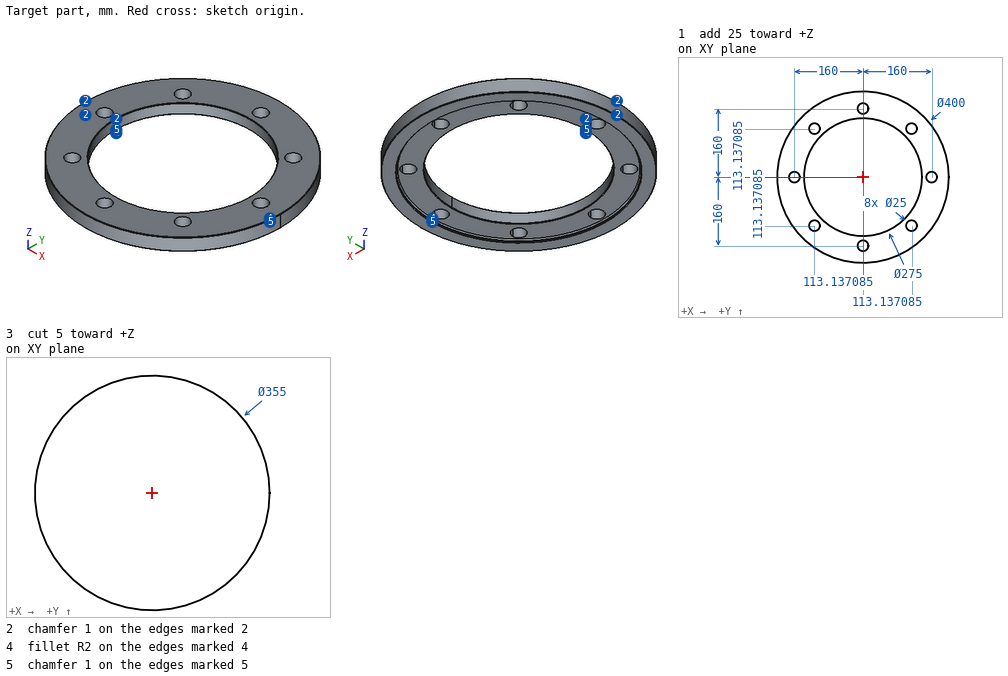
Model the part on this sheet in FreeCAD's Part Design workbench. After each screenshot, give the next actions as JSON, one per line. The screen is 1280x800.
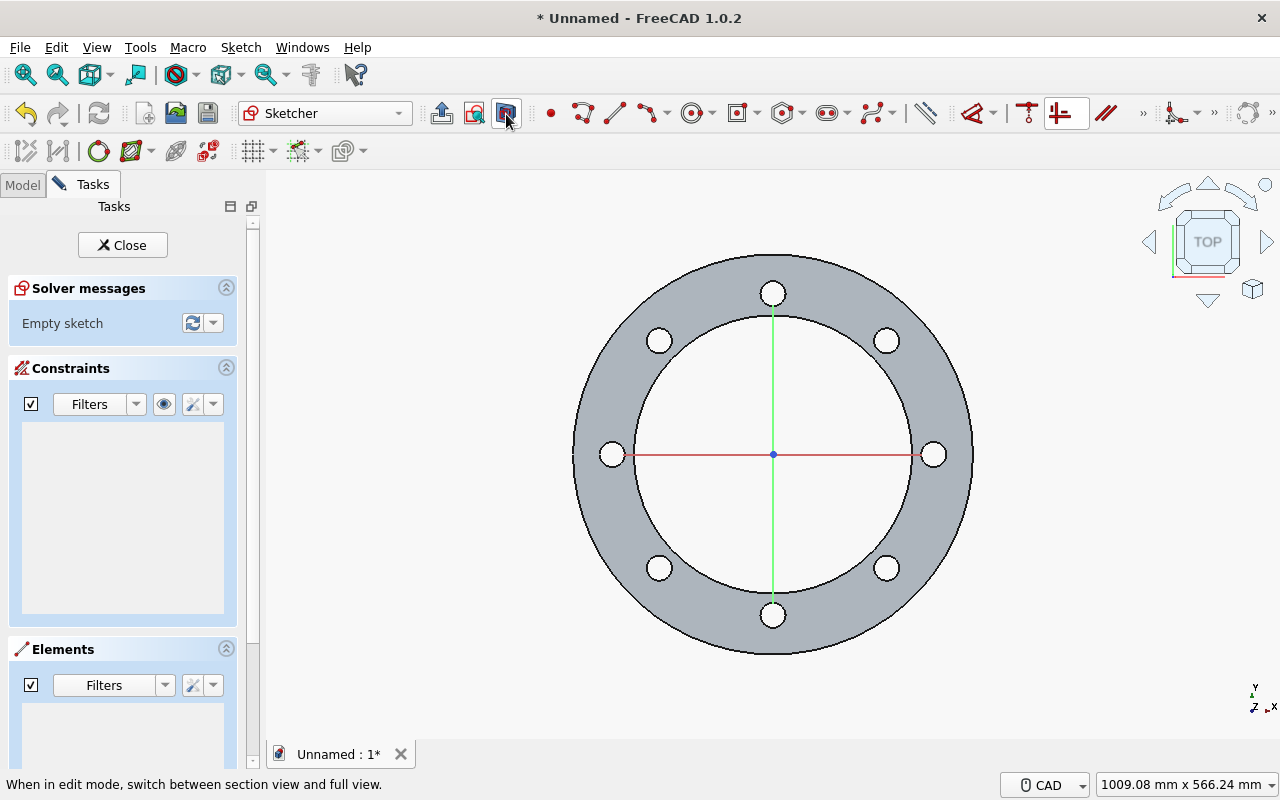
{"action": "left_click", "coordinate": [692, 114]}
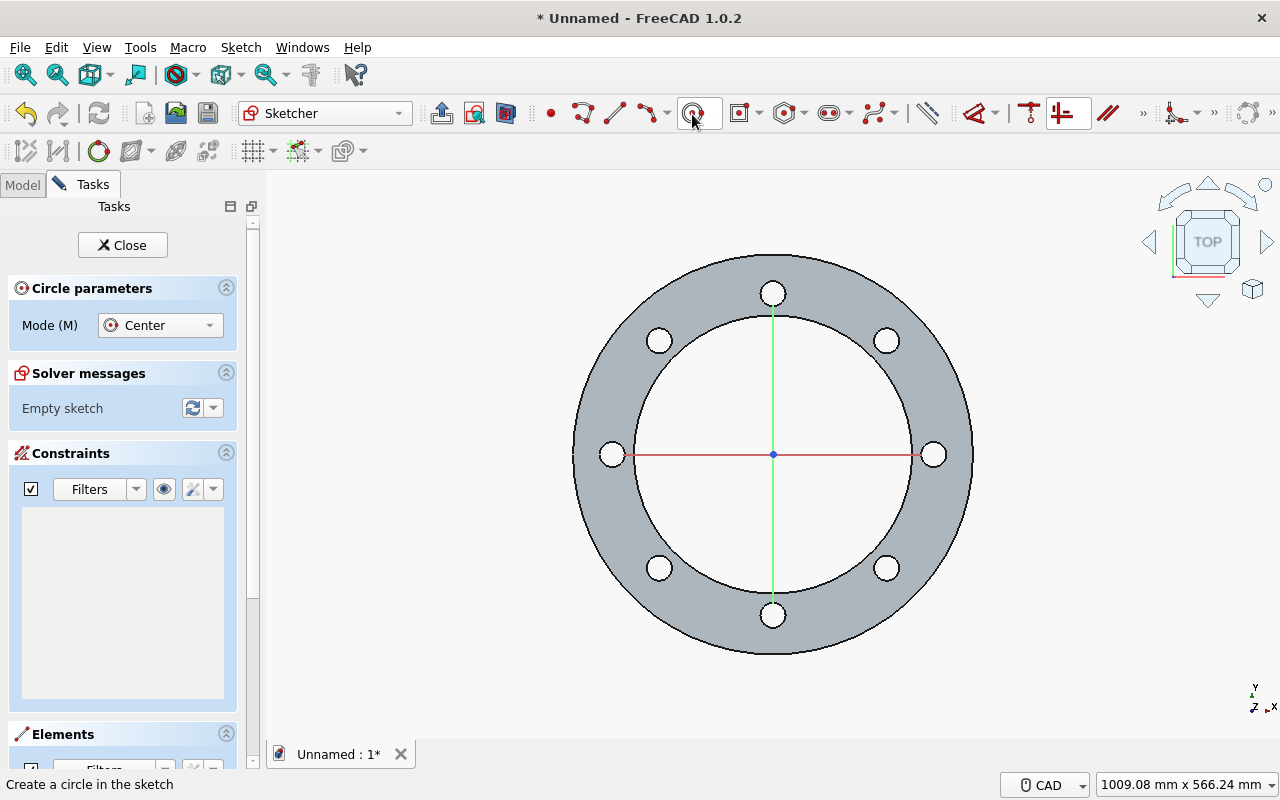
{"action": "left_click", "coordinate": [773, 454]}
{"action": "left_click", "coordinate": [899, 328]}
{"action": "key", "text": "Escape"}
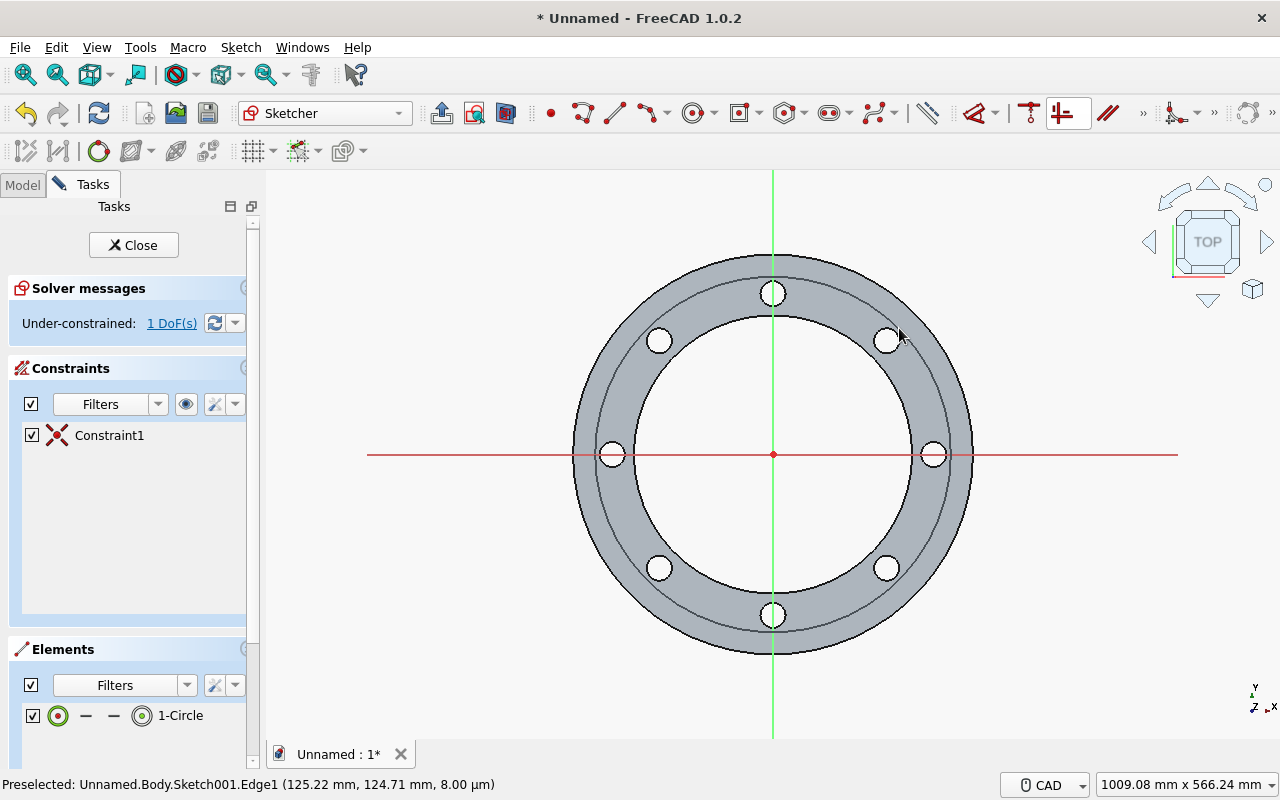
{"action": "left_click", "coordinate": [974, 114]}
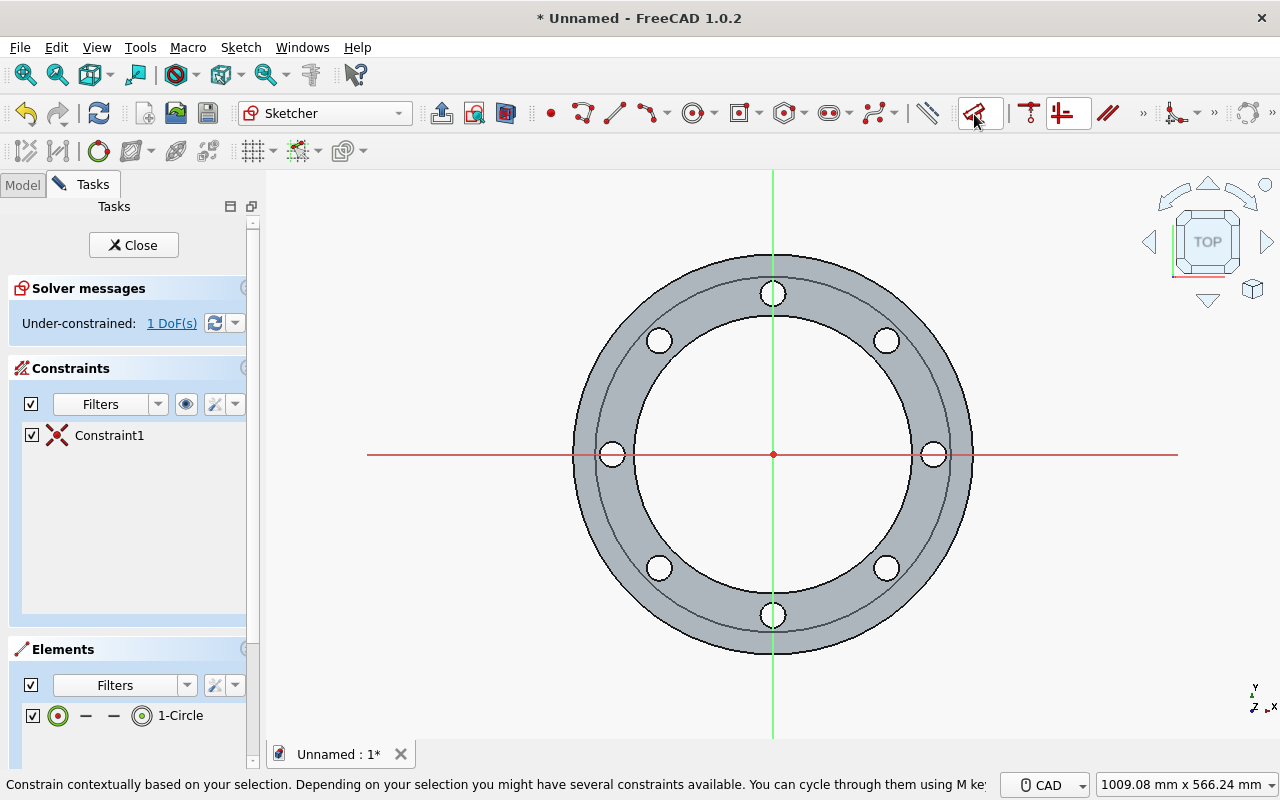
{"action": "left_click", "coordinate": [898, 328]}
{"action": "left_click", "coordinate": [920, 305]}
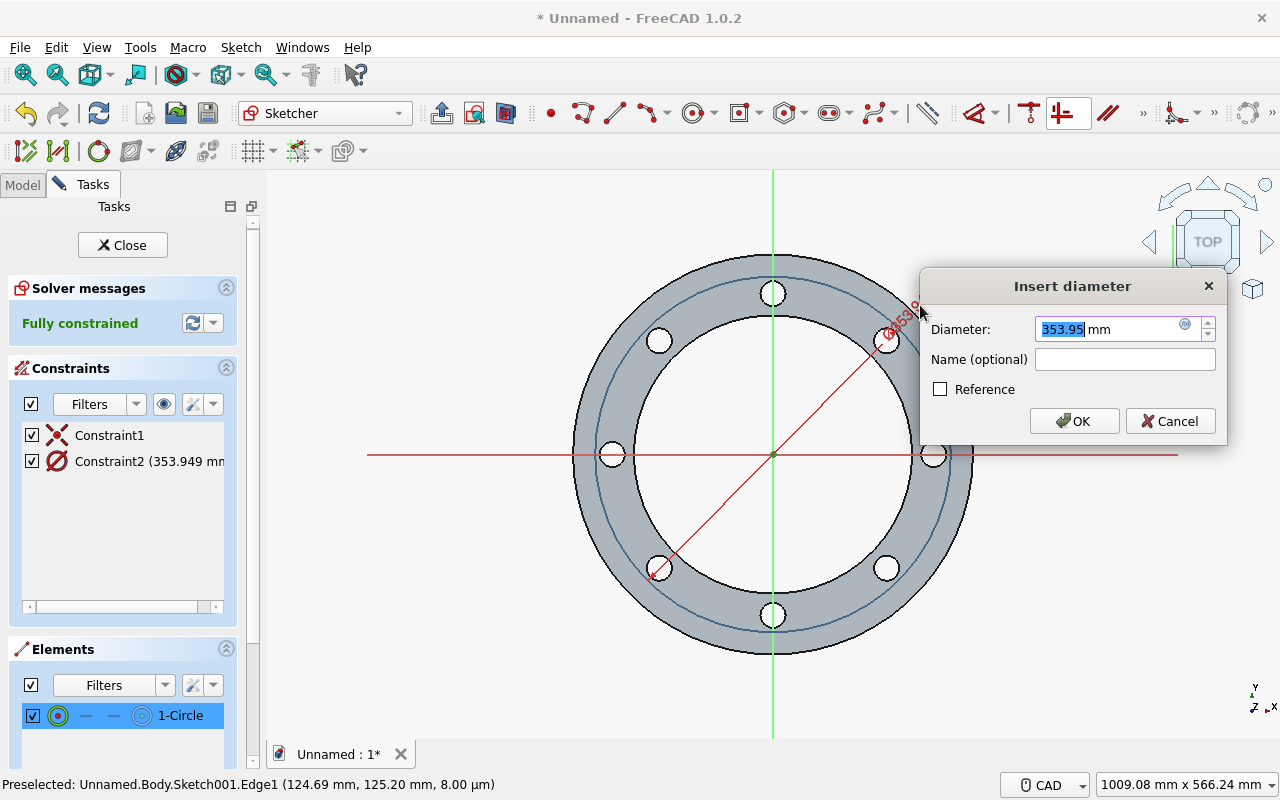
{"action": "type", "text": "355"}
{"action": "key", "text": "Return"}
{"action": "key", "text": "Escape"}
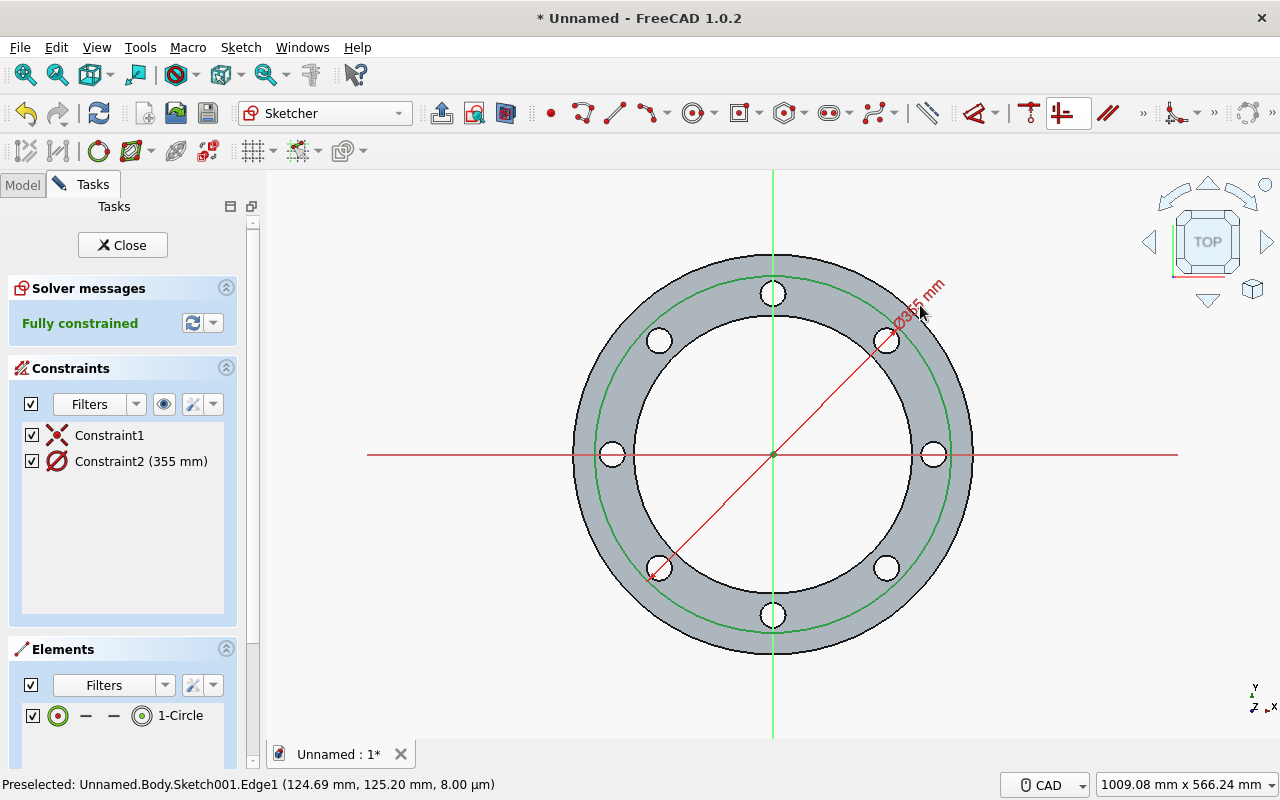
{"action": "left_click", "coordinate": [123, 245]}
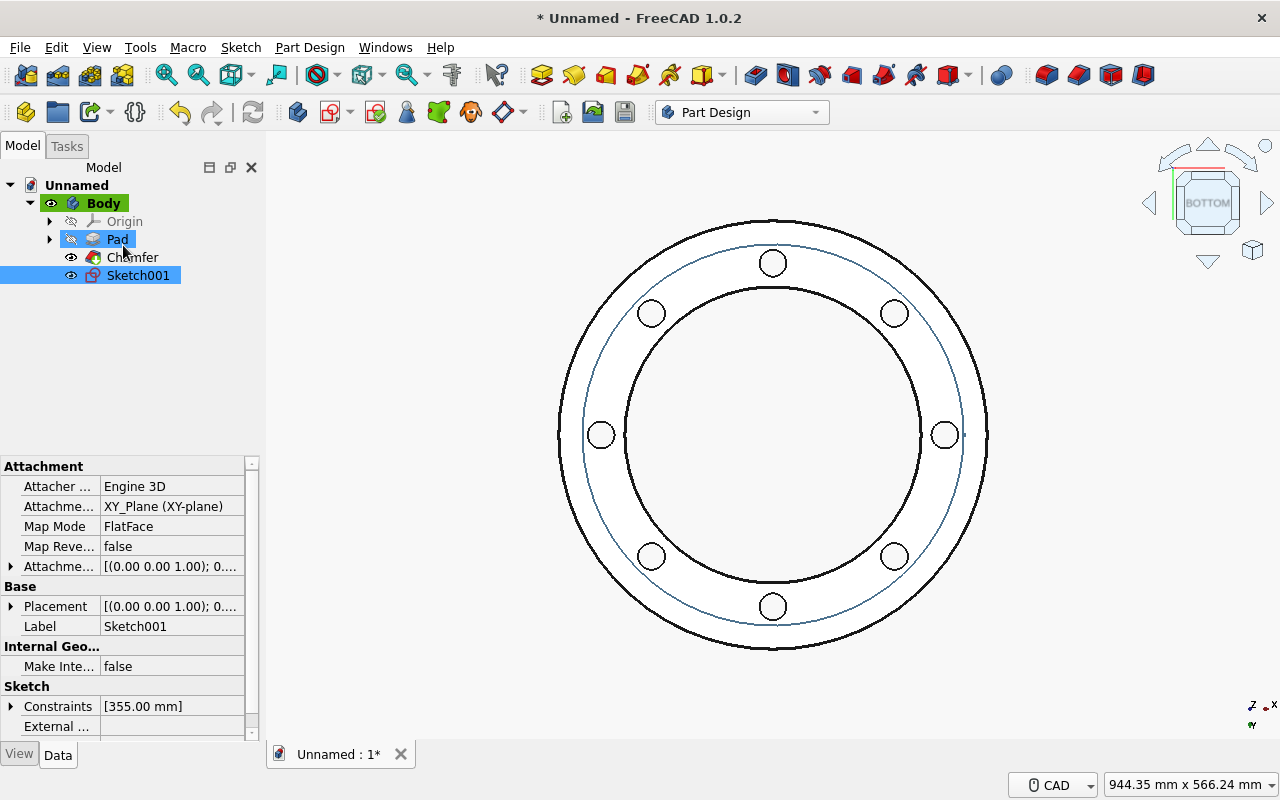
{"action": "left_click", "coordinate": [756, 76]}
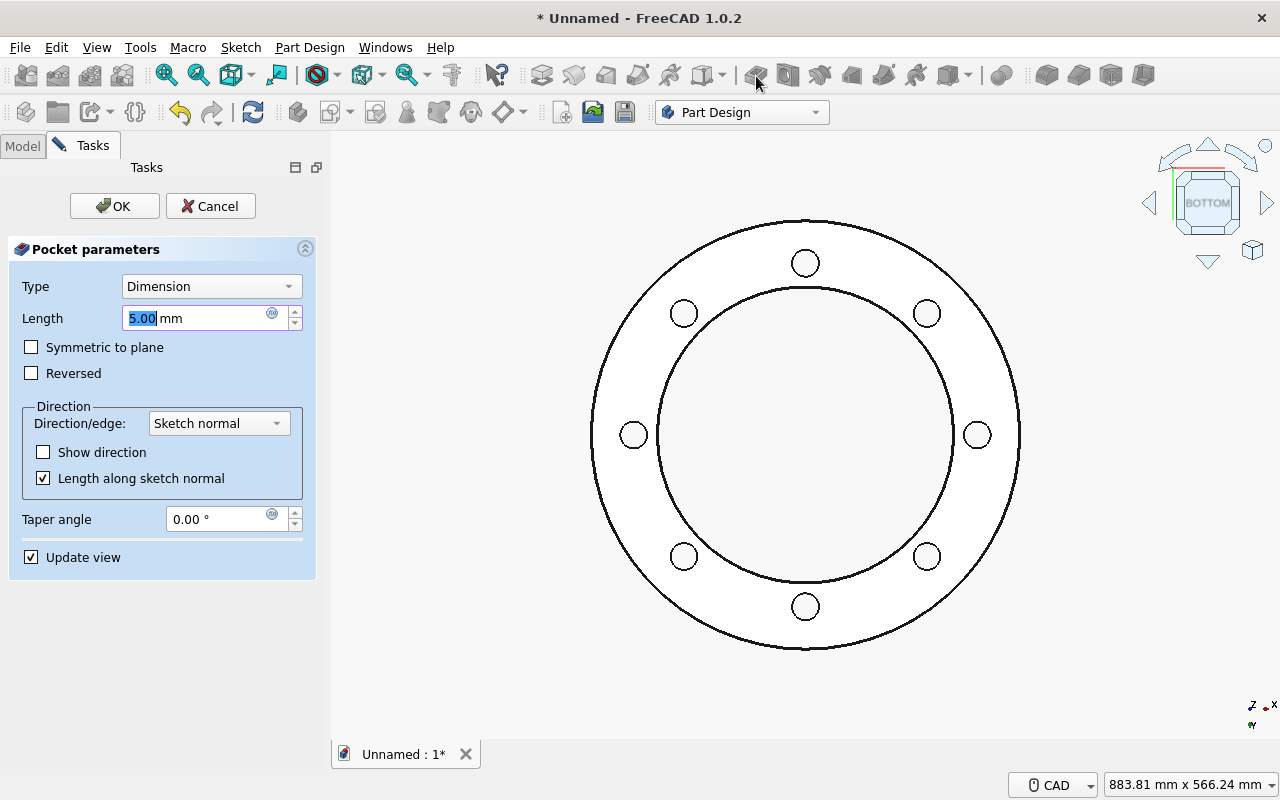
{"action": "type", "text": "5"}
{"action": "key", "text": "Tab"}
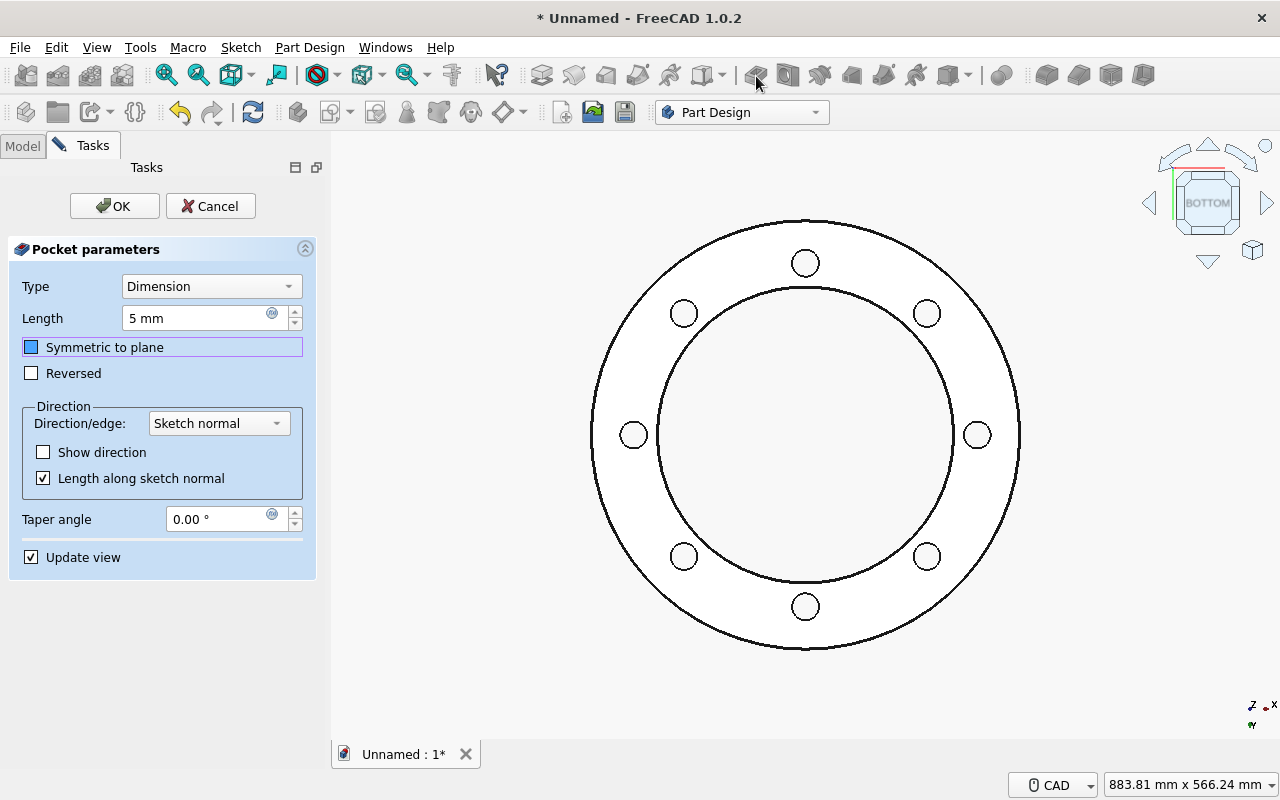
{"action": "left_click", "coordinate": [30, 373]}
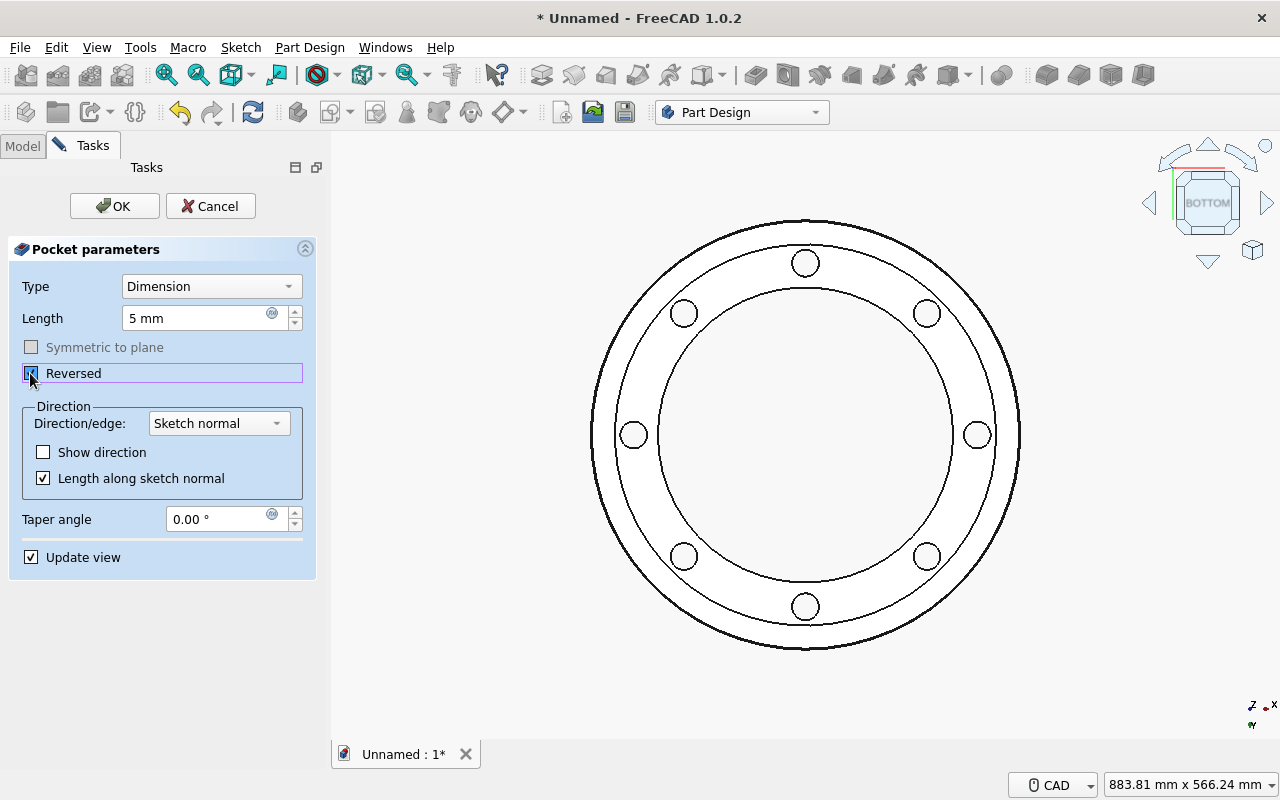
{"action": "left_click", "coordinate": [115, 206]}